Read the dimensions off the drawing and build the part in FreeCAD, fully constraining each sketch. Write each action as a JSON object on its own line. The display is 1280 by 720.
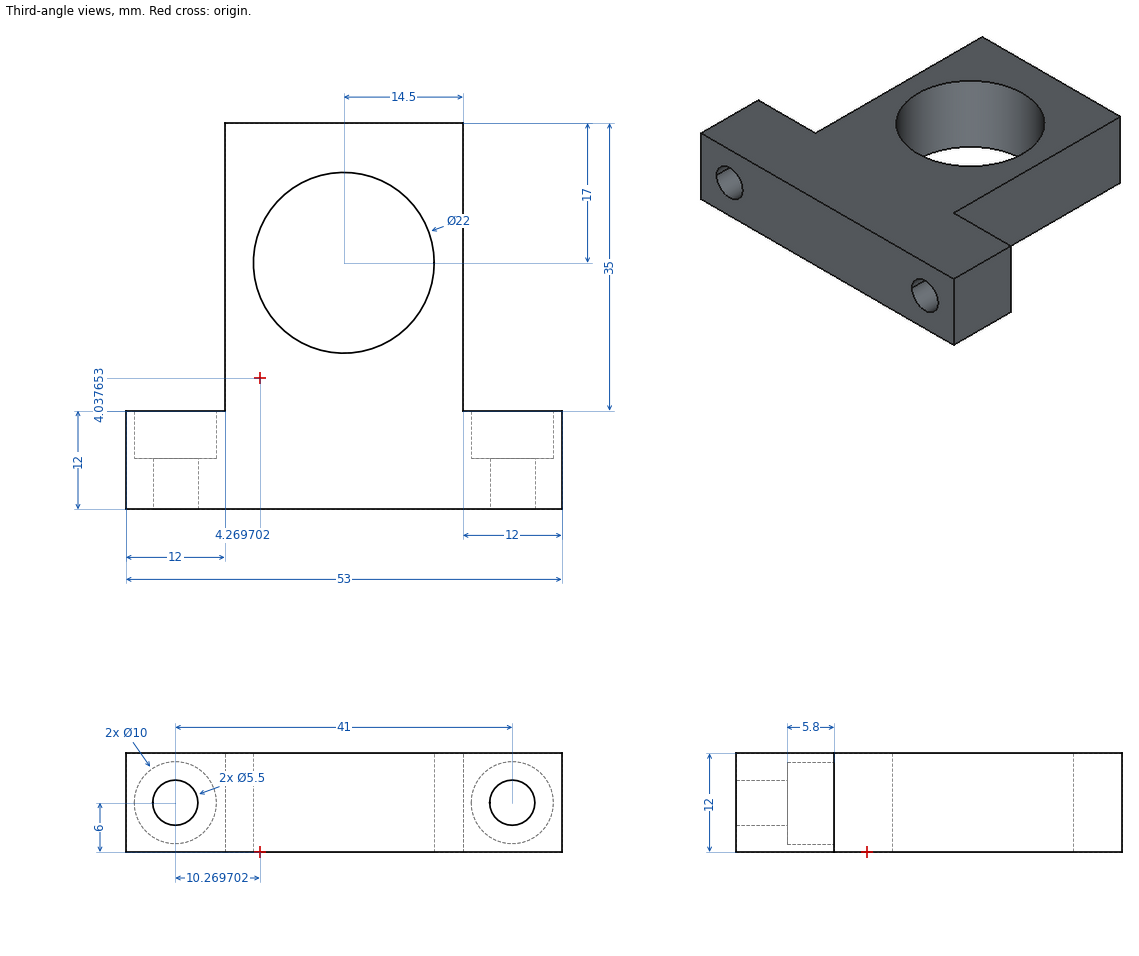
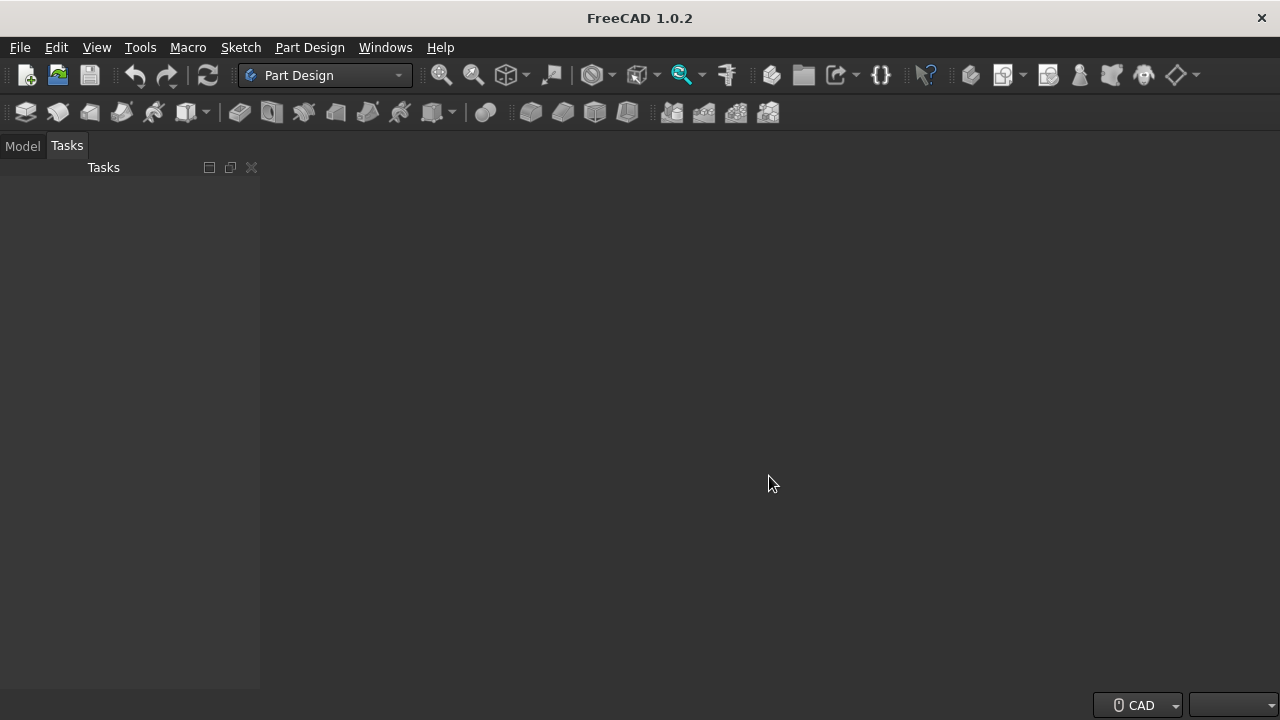
{"action": "key", "text": "ctrl+n"}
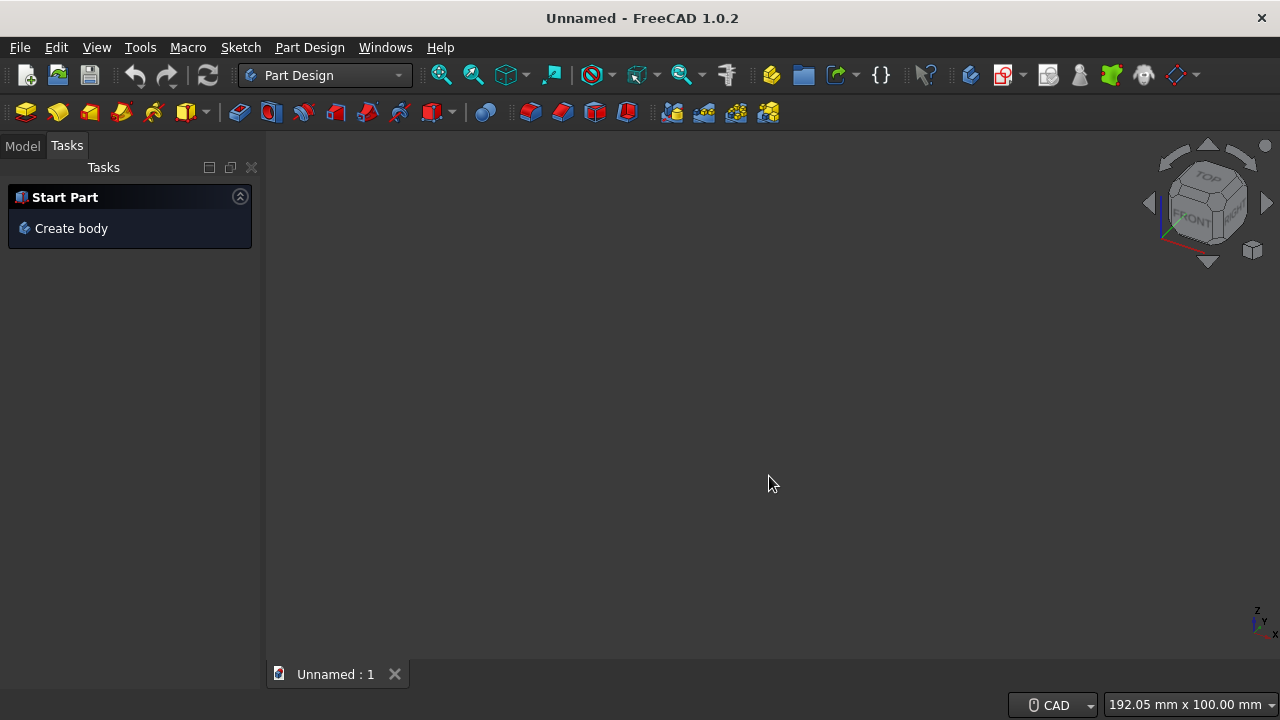
{"action": "left_click", "coordinate": [1004, 76]}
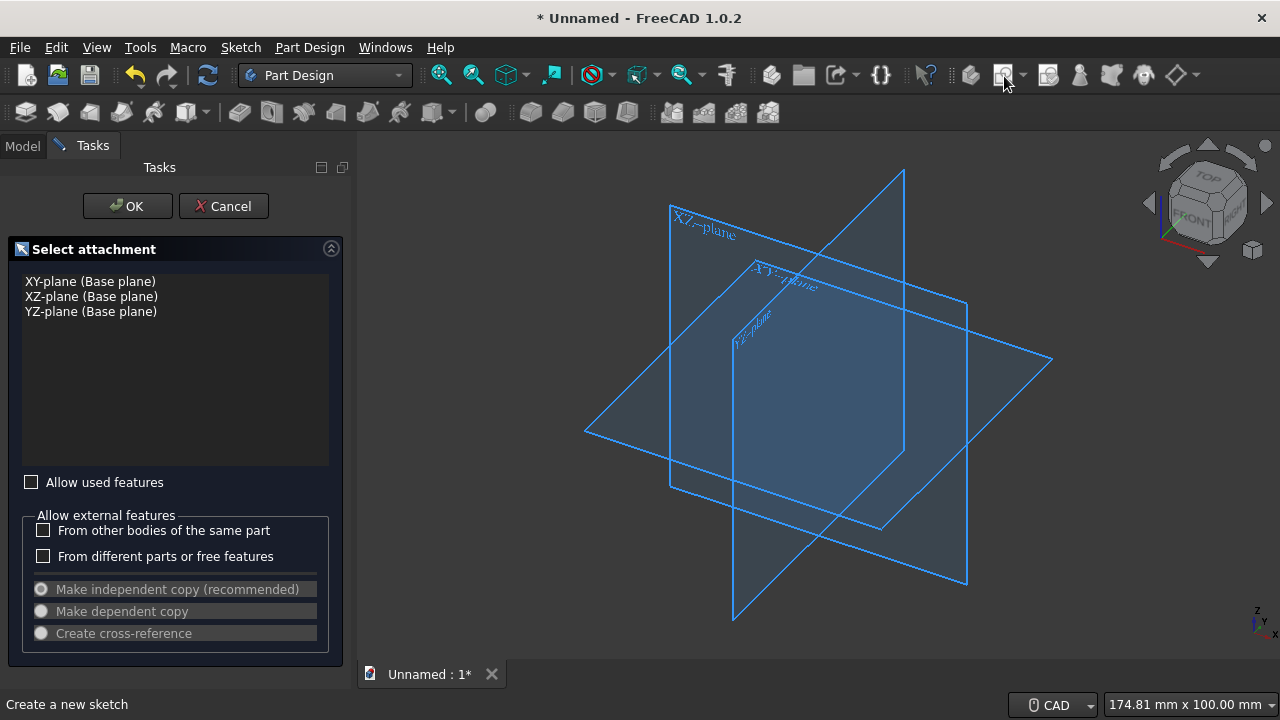
{"action": "left_click", "coordinate": [82, 282]}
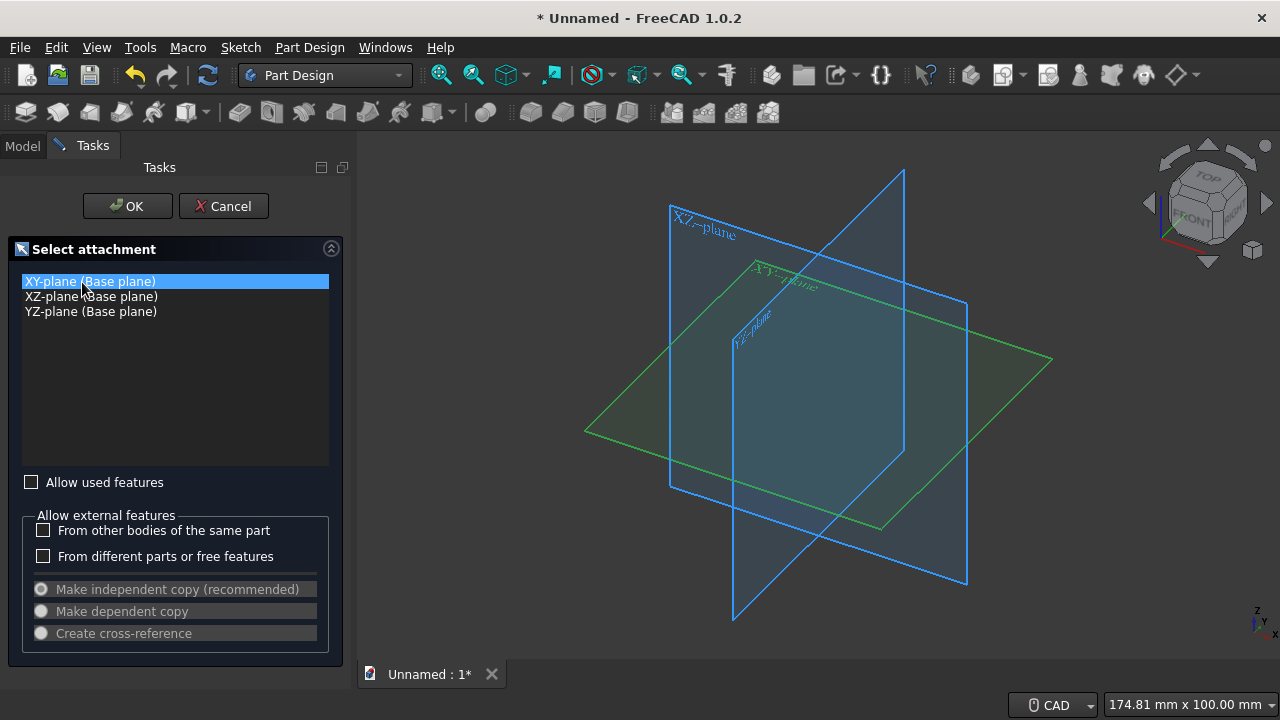
{"action": "left_click", "coordinate": [128, 206]}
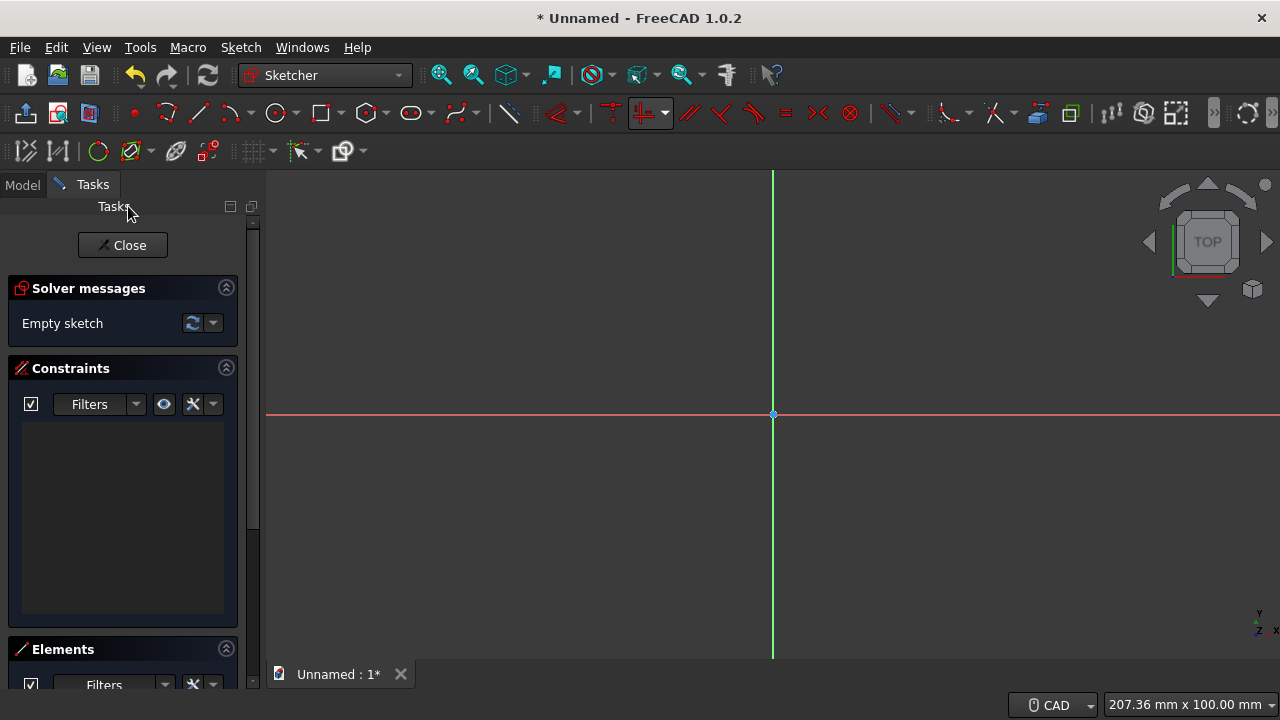
{"action": "left_click", "coordinate": [168, 114]}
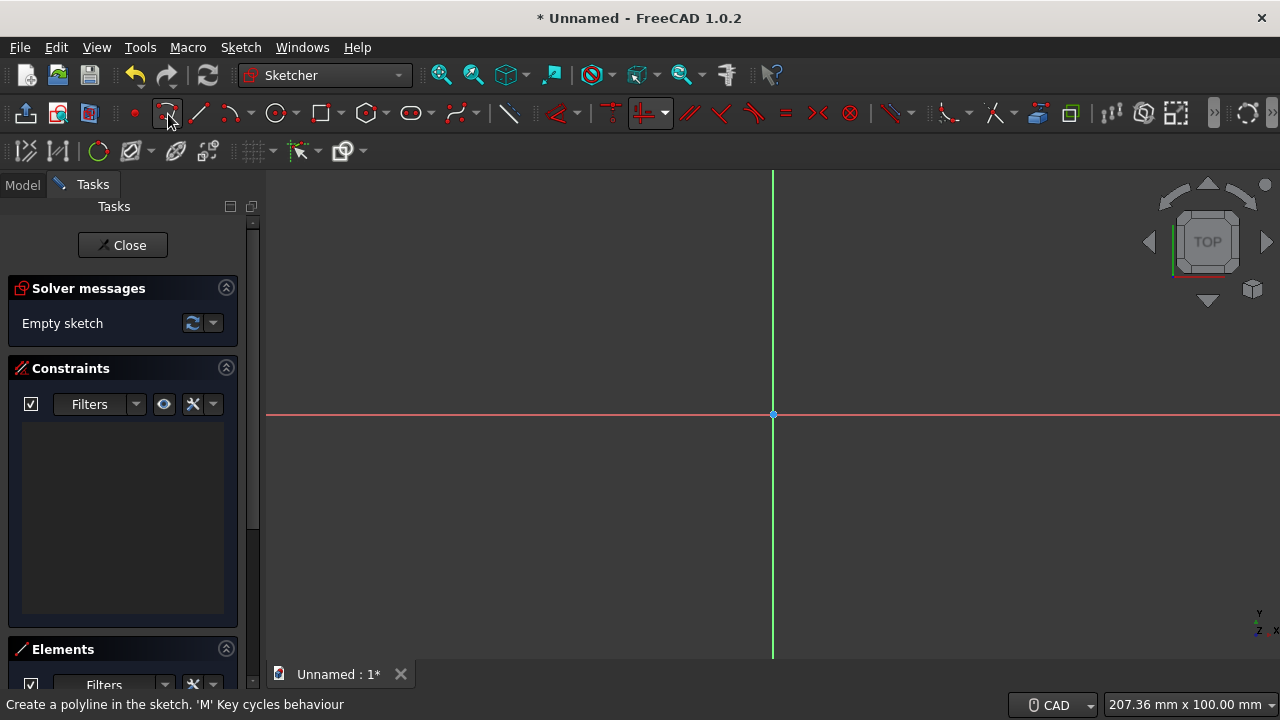
{"action": "left_click", "coordinate": [752, 434]}
{"action": "left_click", "coordinate": [693, 434]}
{"action": "left_click", "coordinate": [693, 493]}
{"action": "left_click", "coordinate": [953, 493]}
{"action": "left_click", "coordinate": [953, 434]}
{"action": "left_click", "coordinate": [894, 434]}
{"action": "left_click", "coordinate": [894, 263]}
{"action": "left_click", "coordinate": [752, 263]}
{"action": "left_click", "coordinate": [752, 435]}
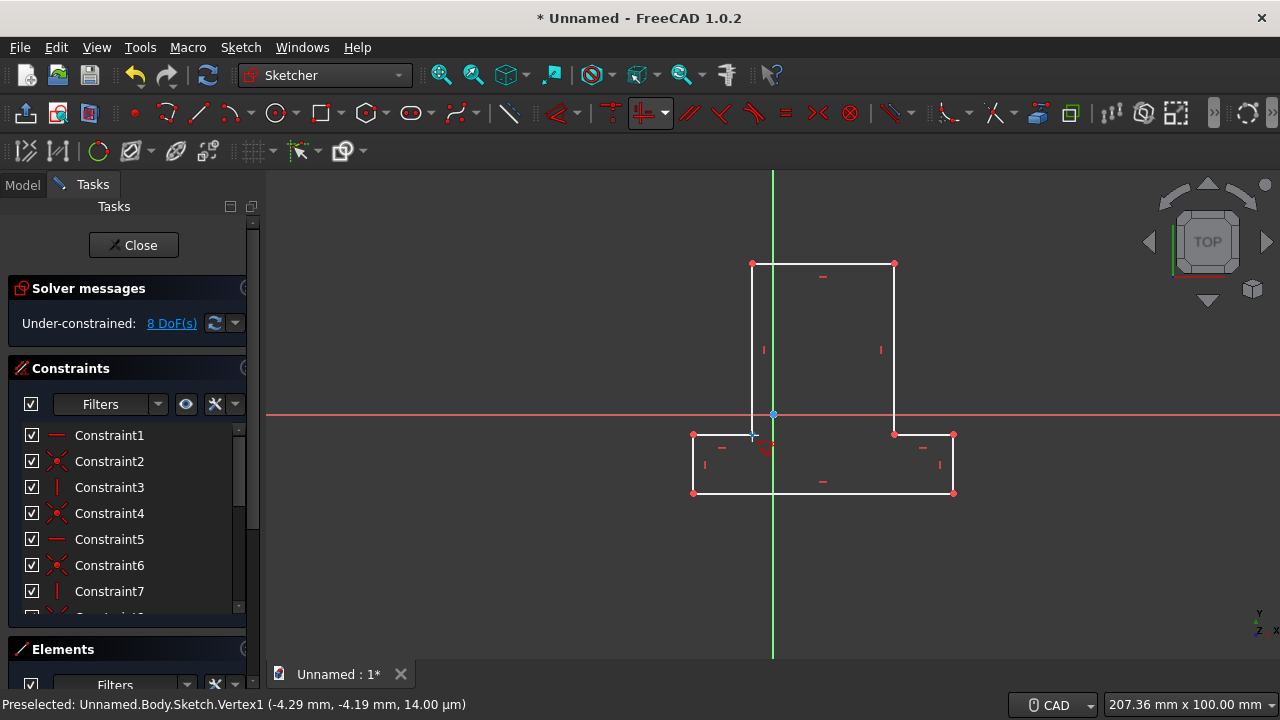
{"action": "left_click", "coordinate": [276, 114]}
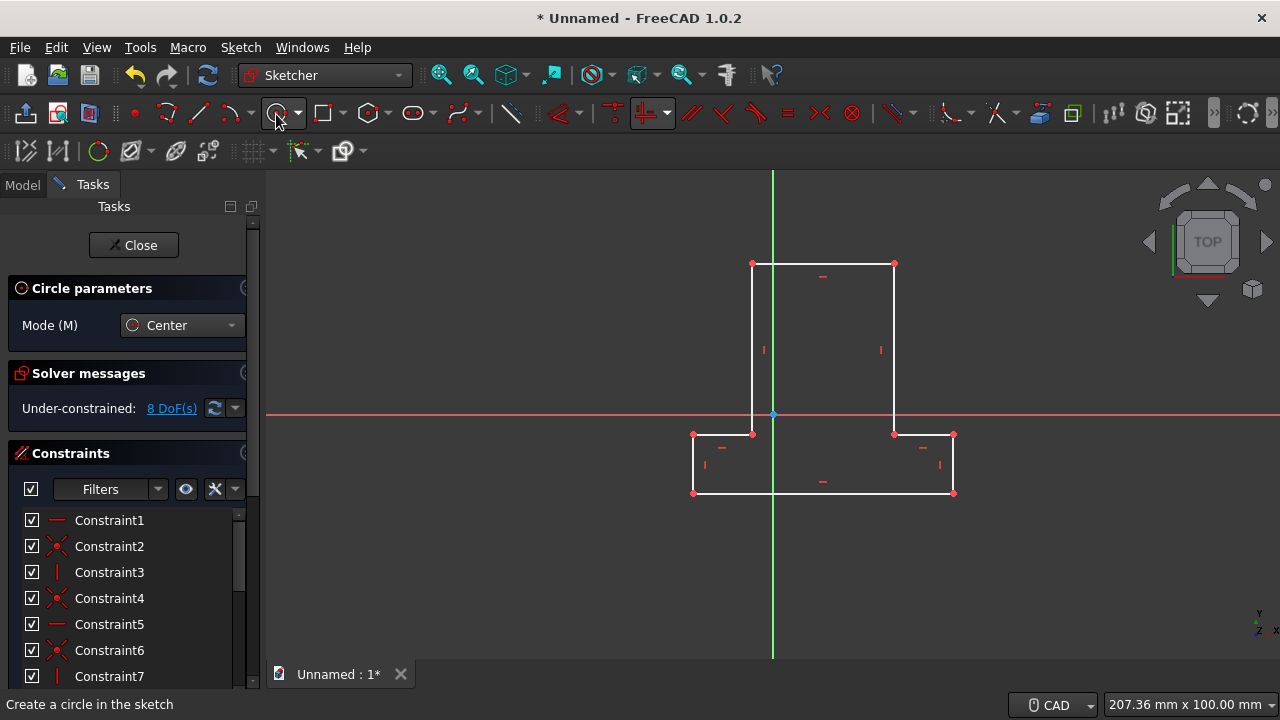
{"action": "left_click", "coordinate": [823, 346]}
{"action": "mouse_move", "coordinate": [861, 308]}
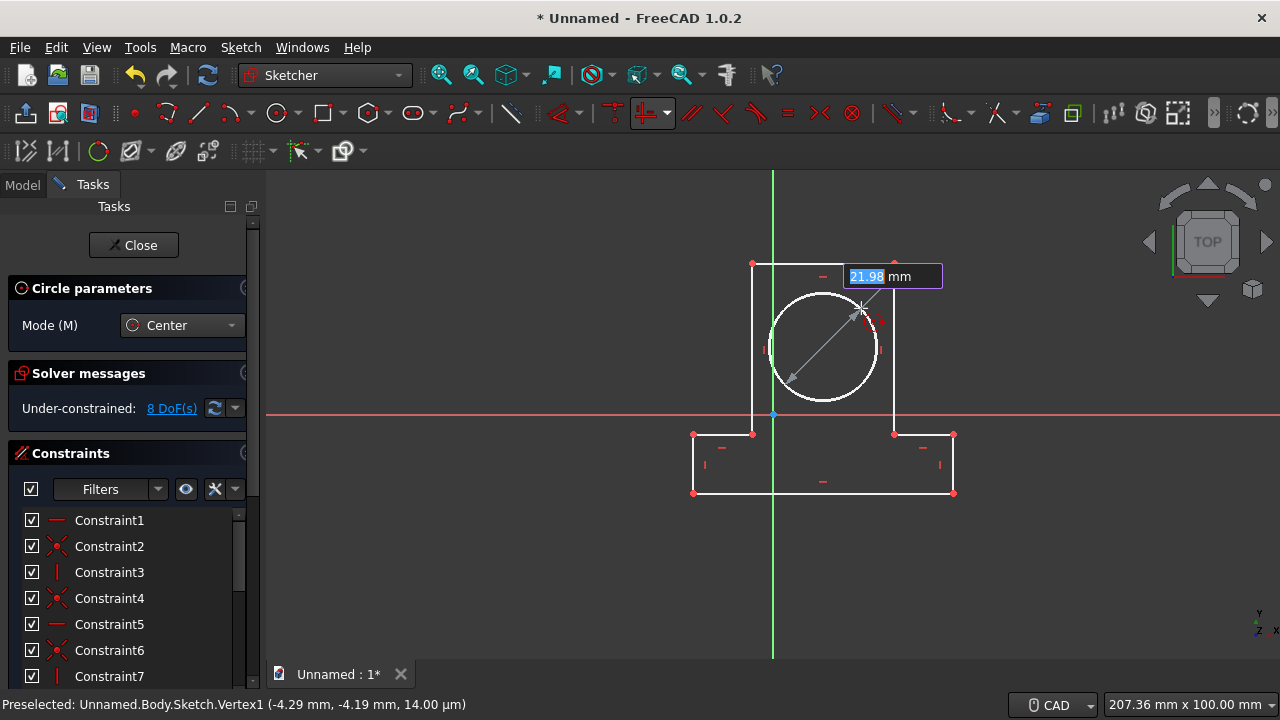
{"action": "type", "text": "22"}
{"action": "key", "text": "Return"}
{"action": "key", "text": "Escape"}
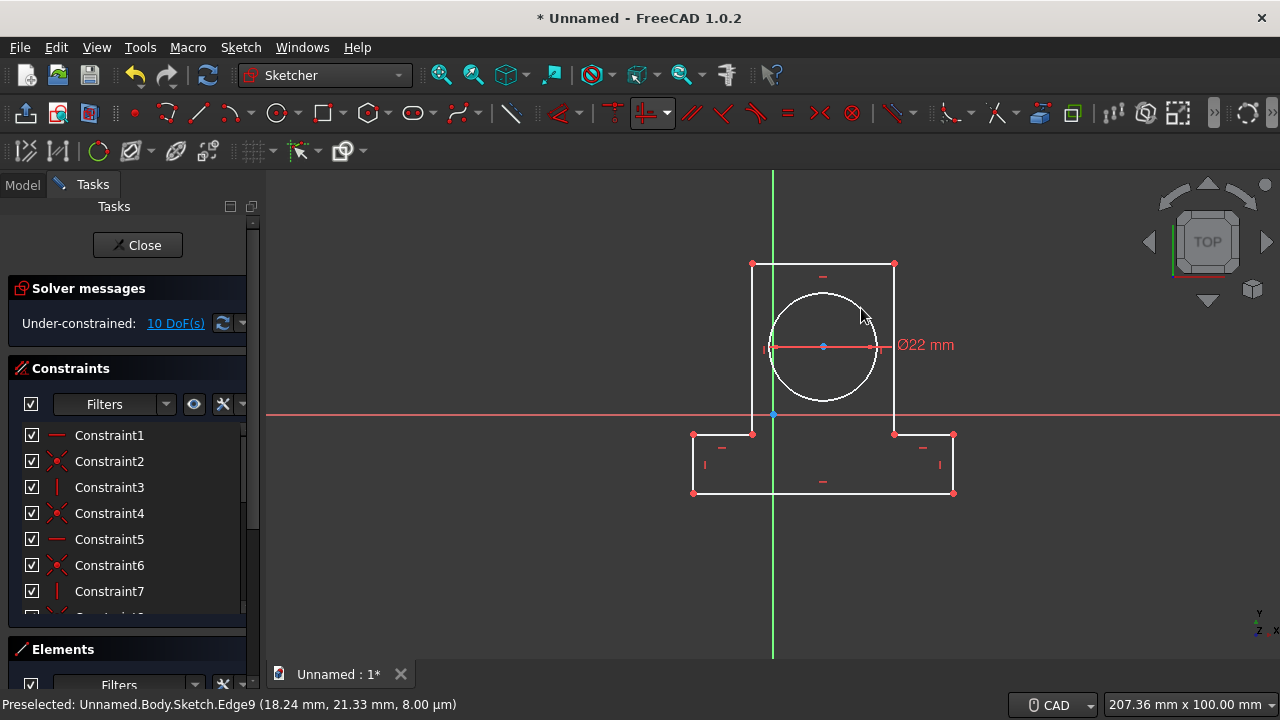
{"action": "left_click", "coordinate": [558, 114]}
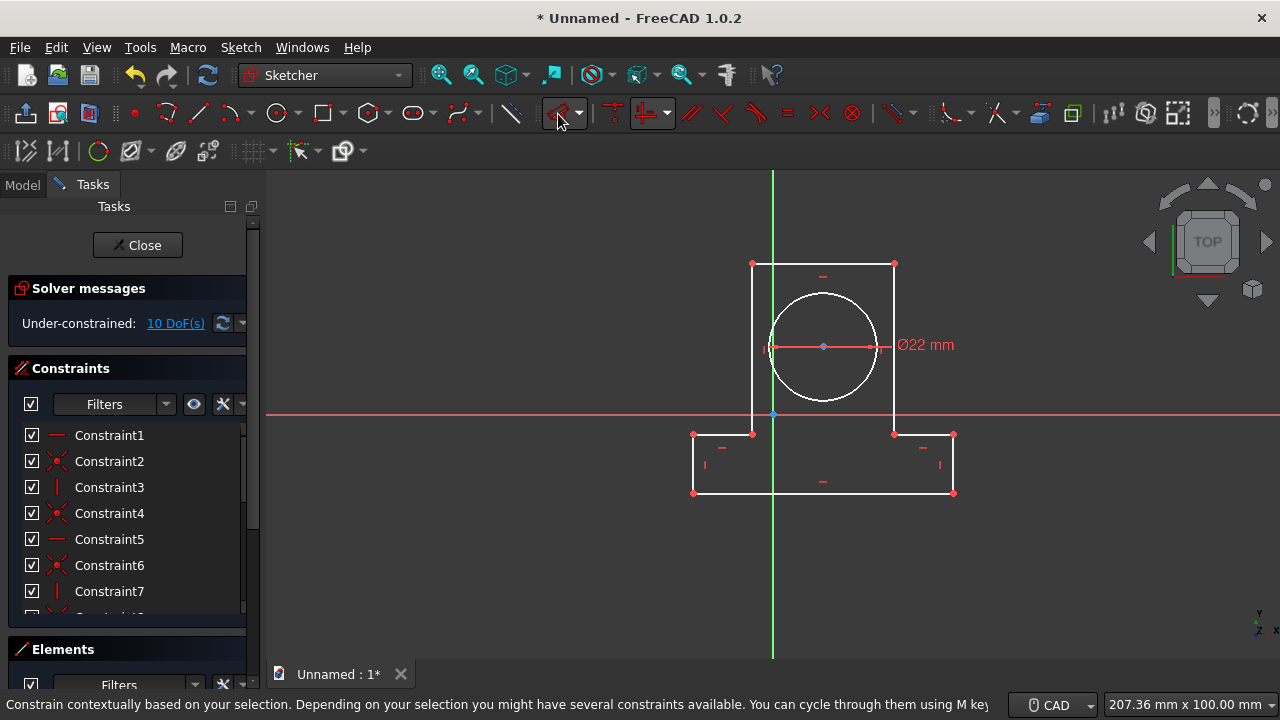
{"action": "left_click", "coordinate": [734, 435]}
{"action": "left_click", "coordinate": [723, 469]}